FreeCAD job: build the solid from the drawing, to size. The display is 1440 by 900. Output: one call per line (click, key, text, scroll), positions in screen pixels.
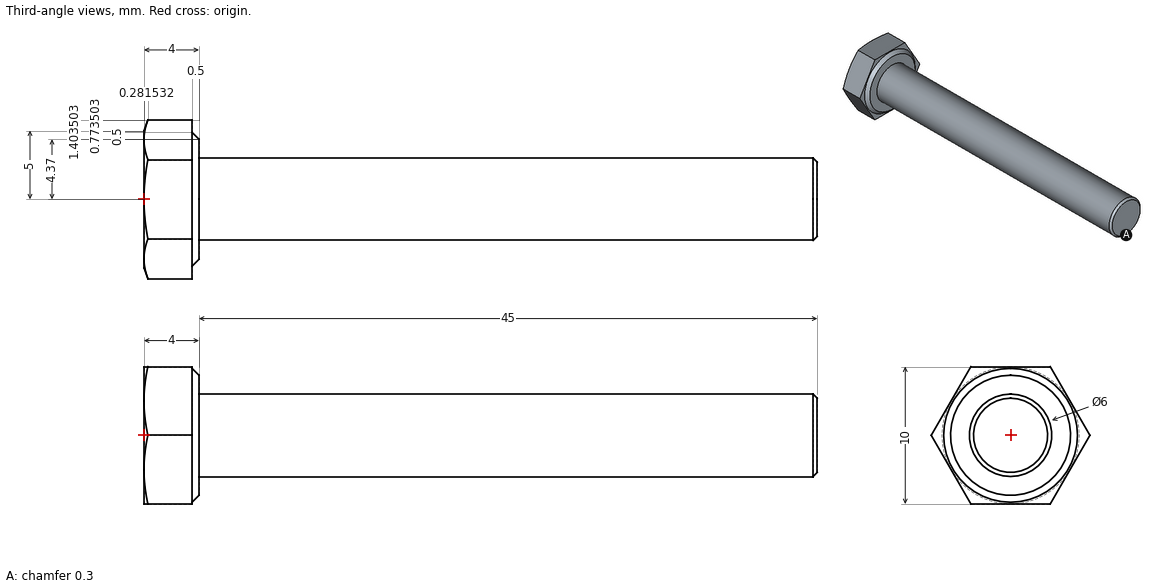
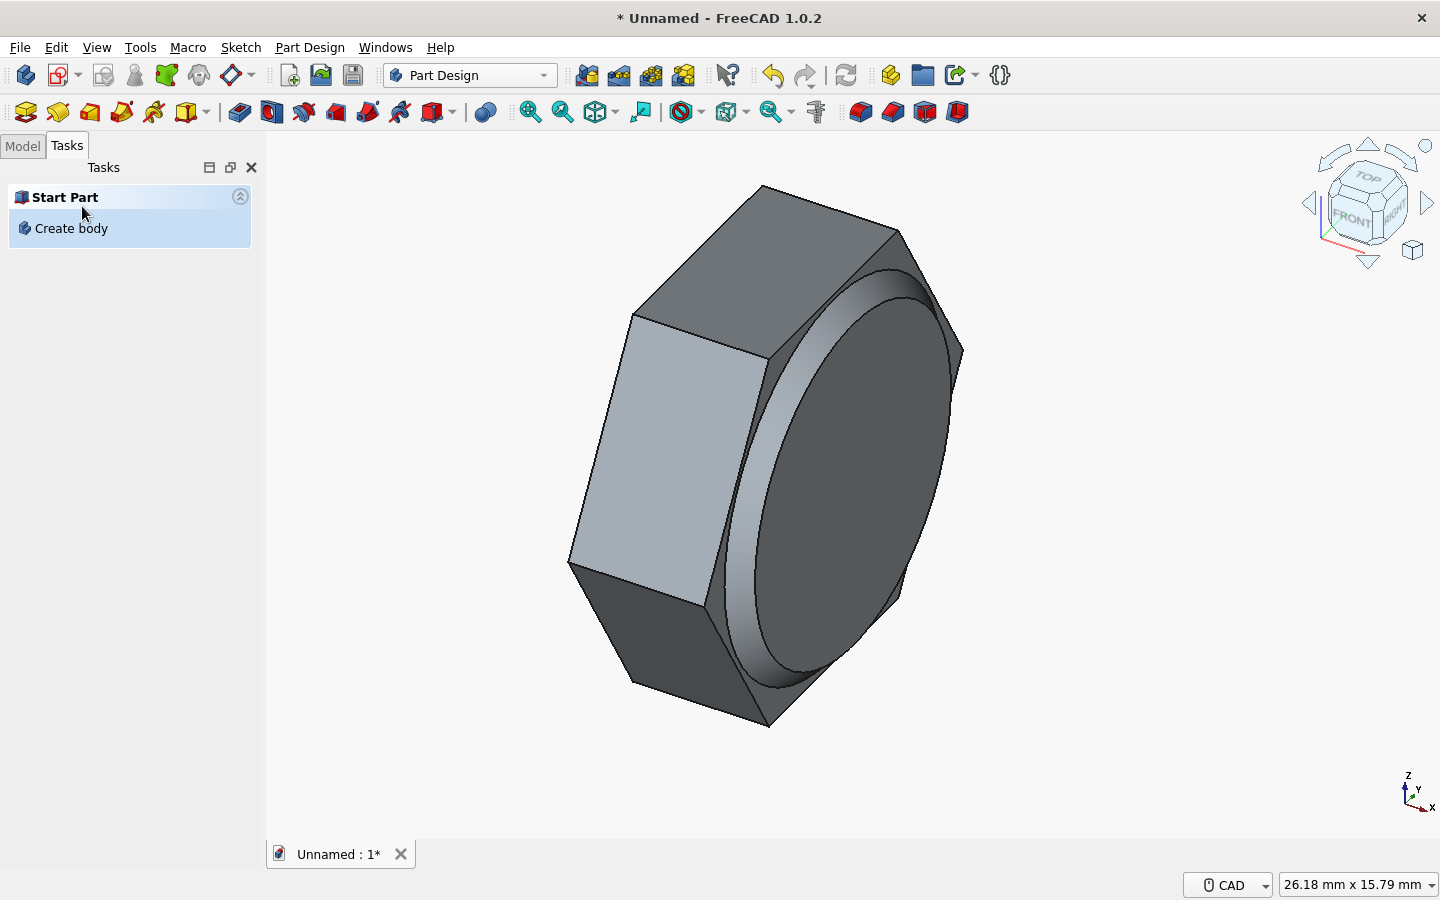
click(532, 112)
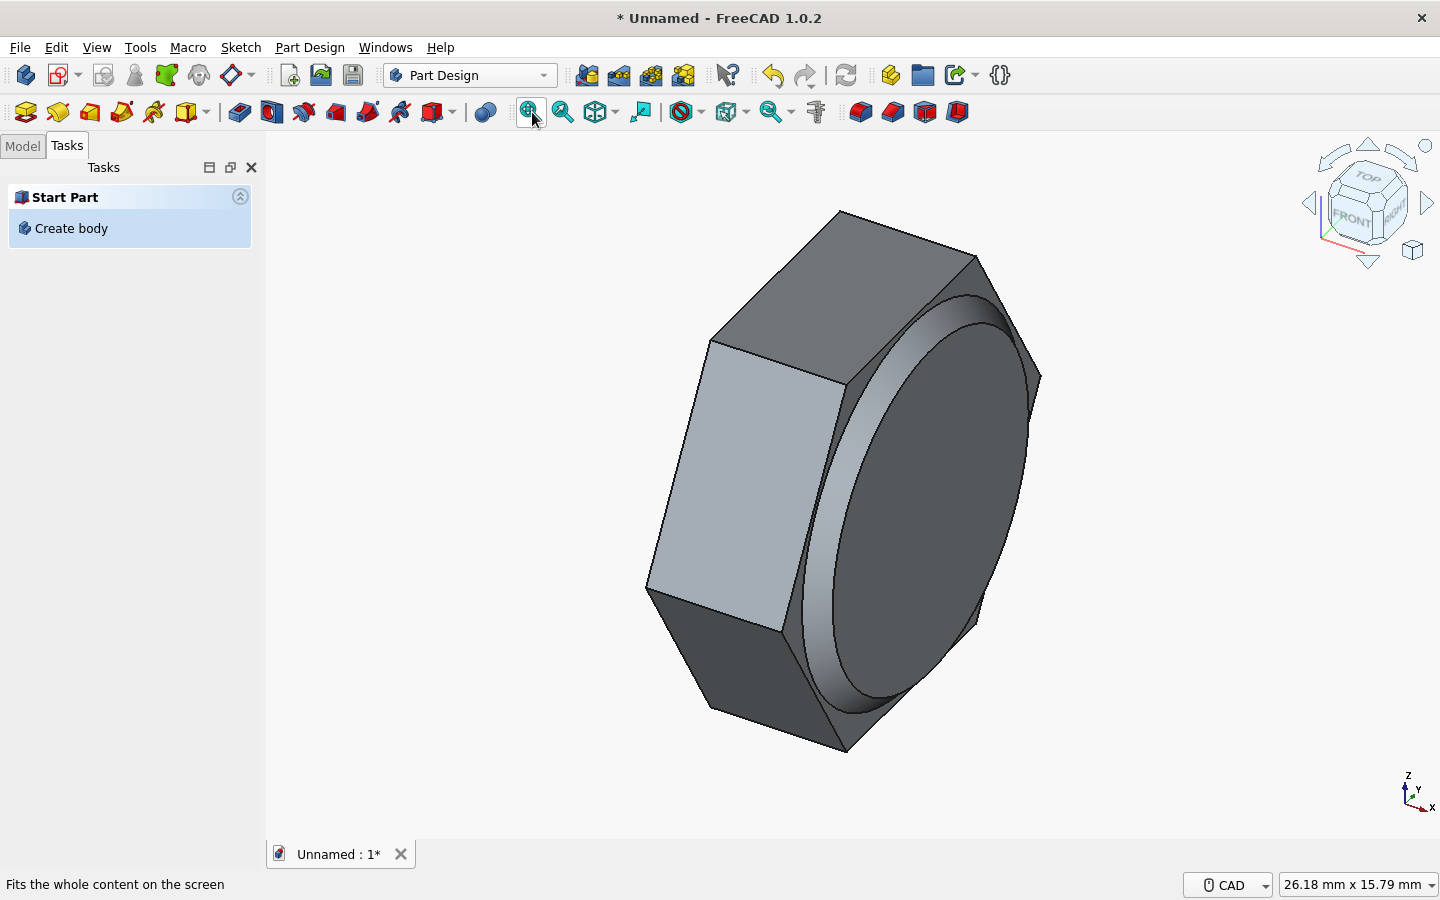
click(58, 76)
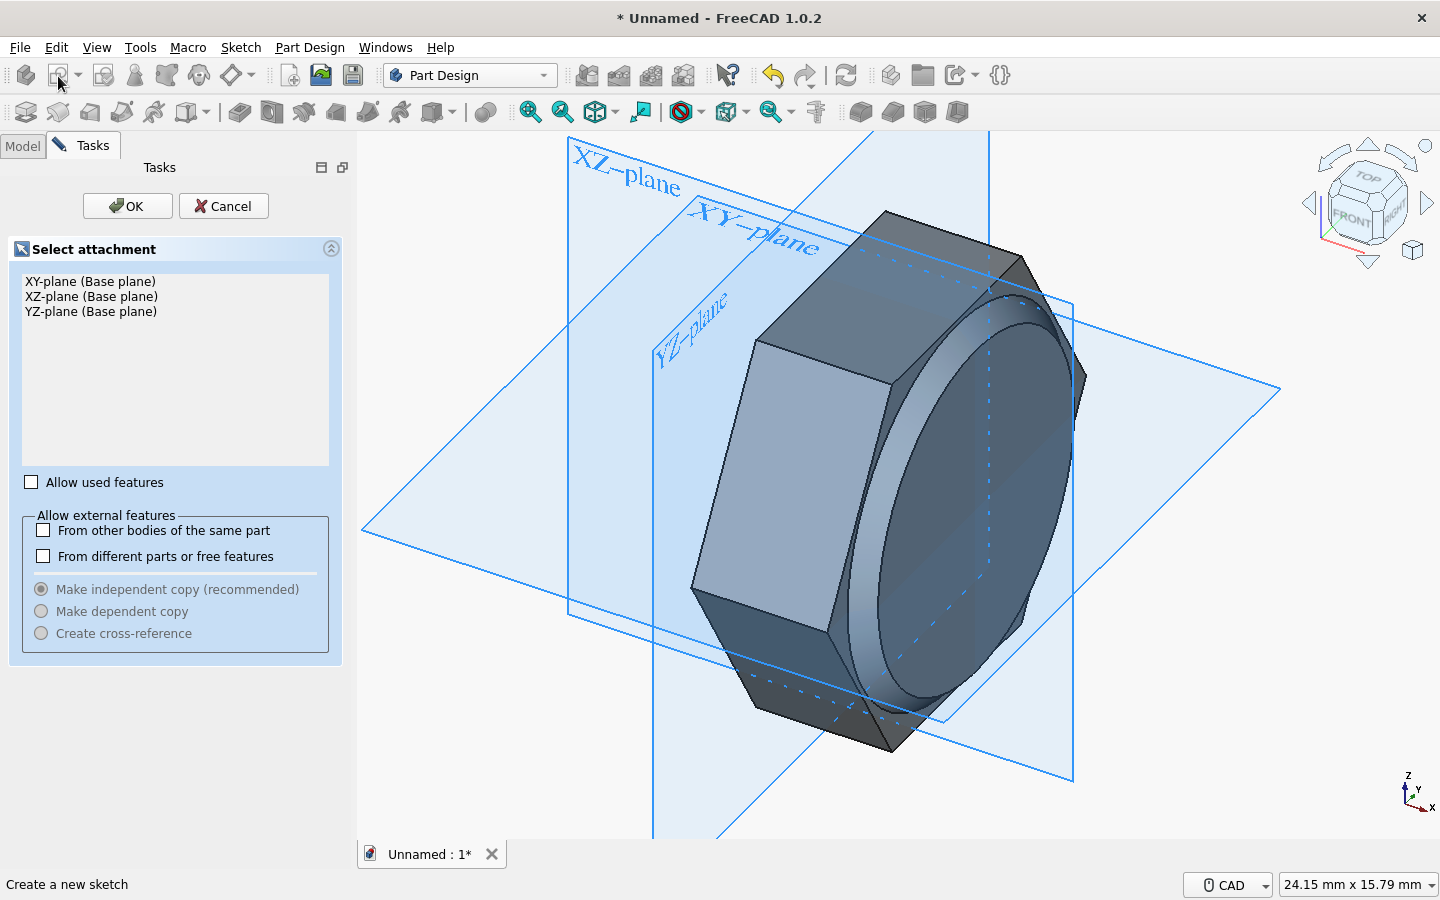
click(82, 282)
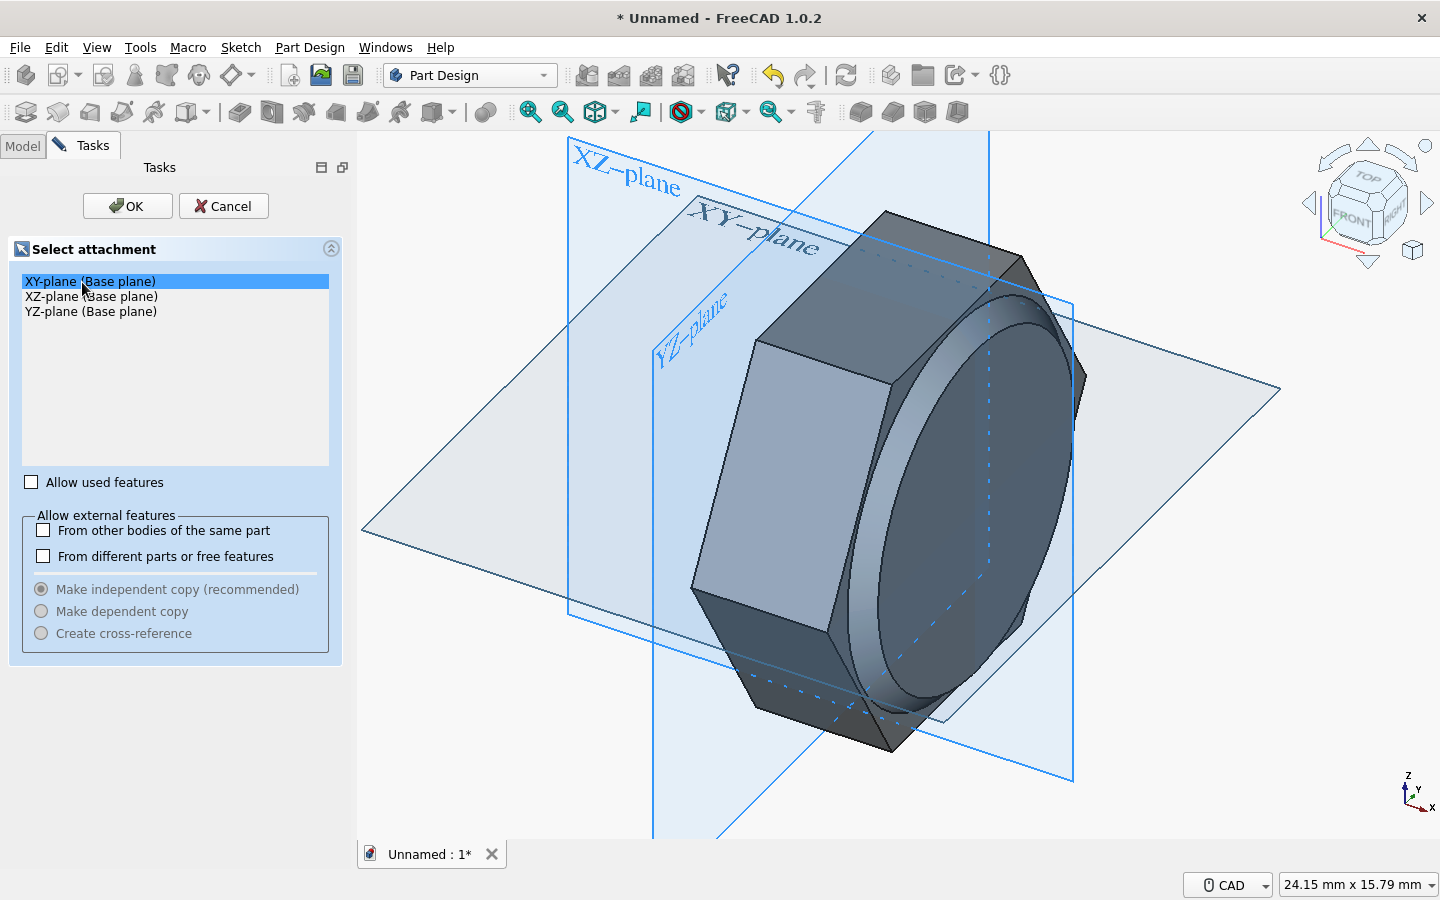
click(128, 206)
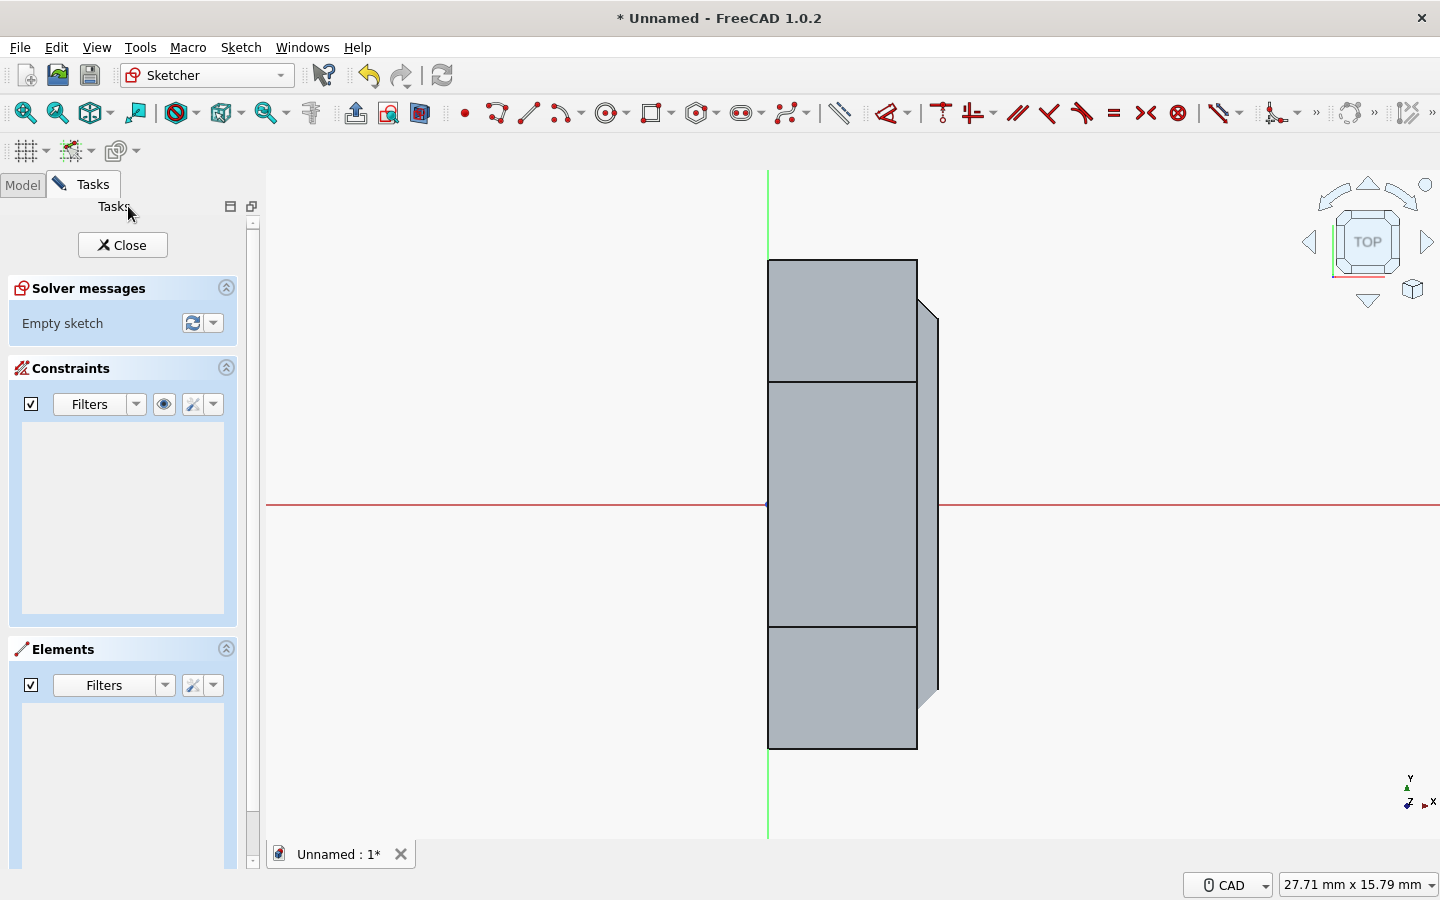
click(420, 114)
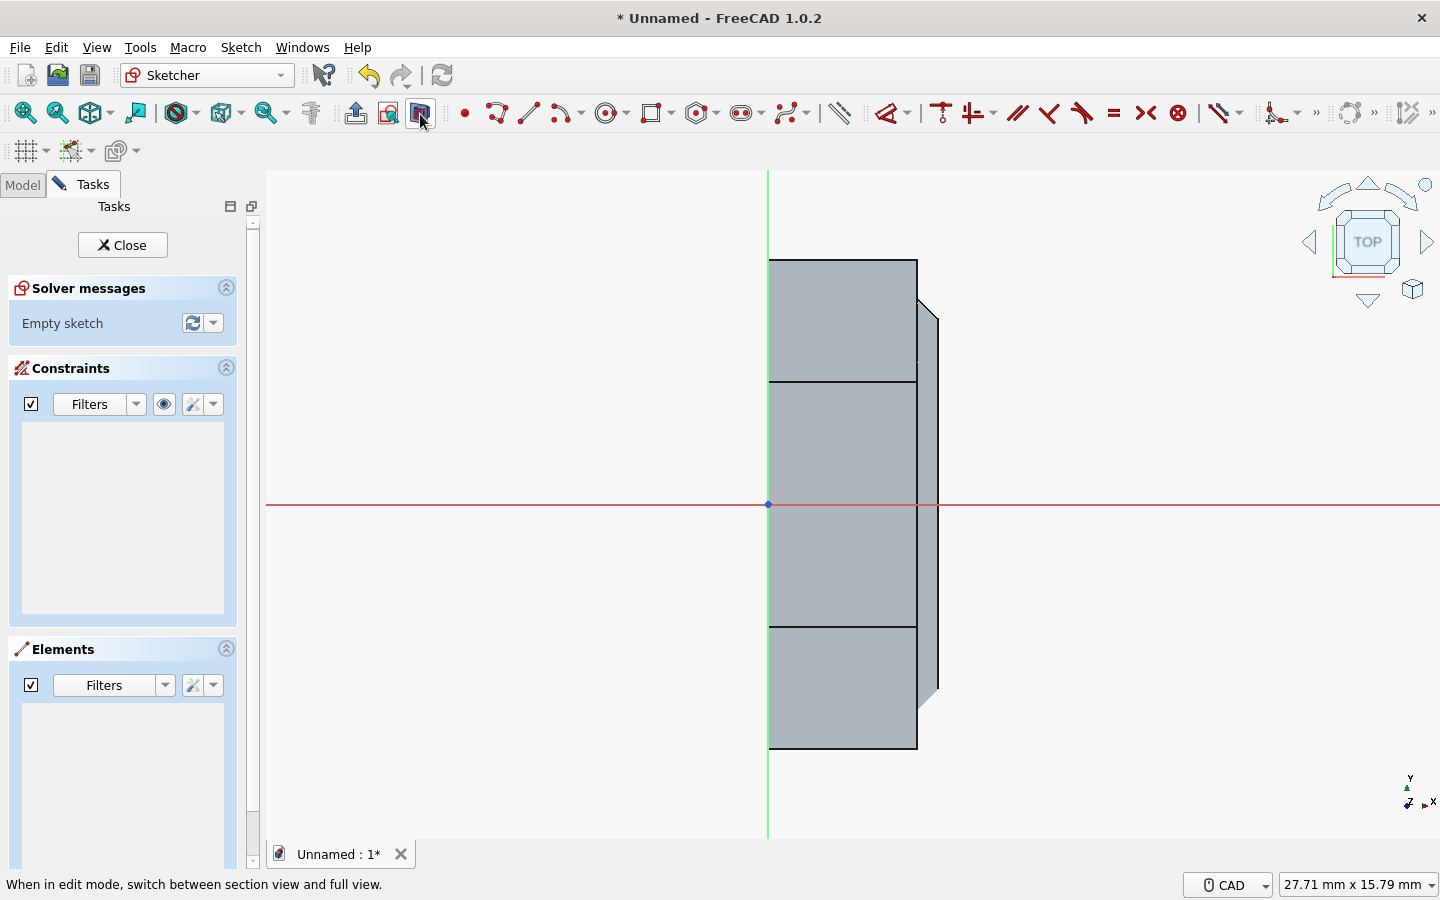
scroll(773, 258, up, 13)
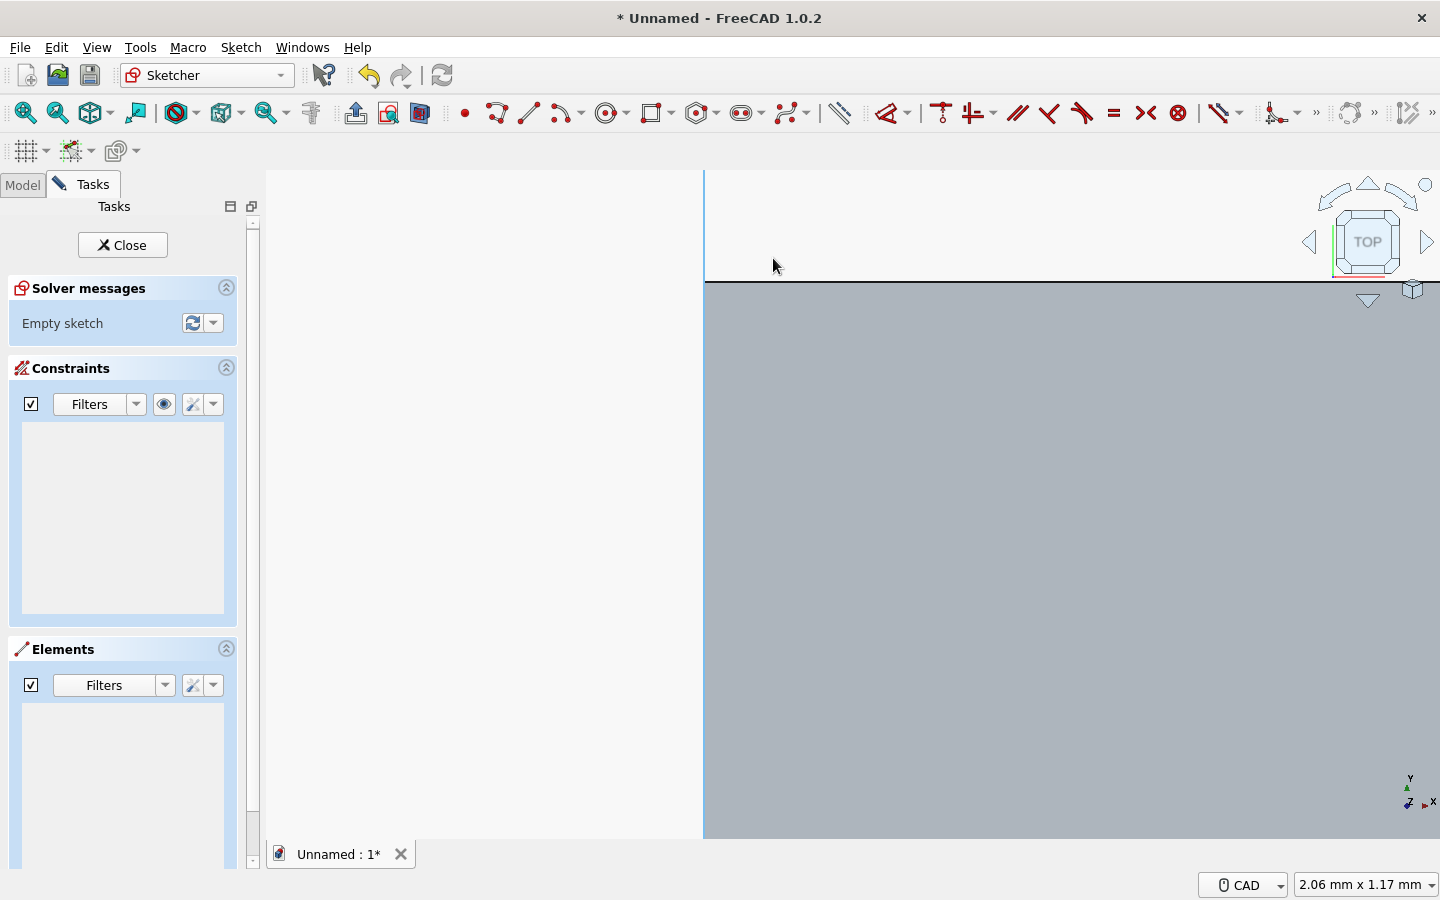
click(498, 114)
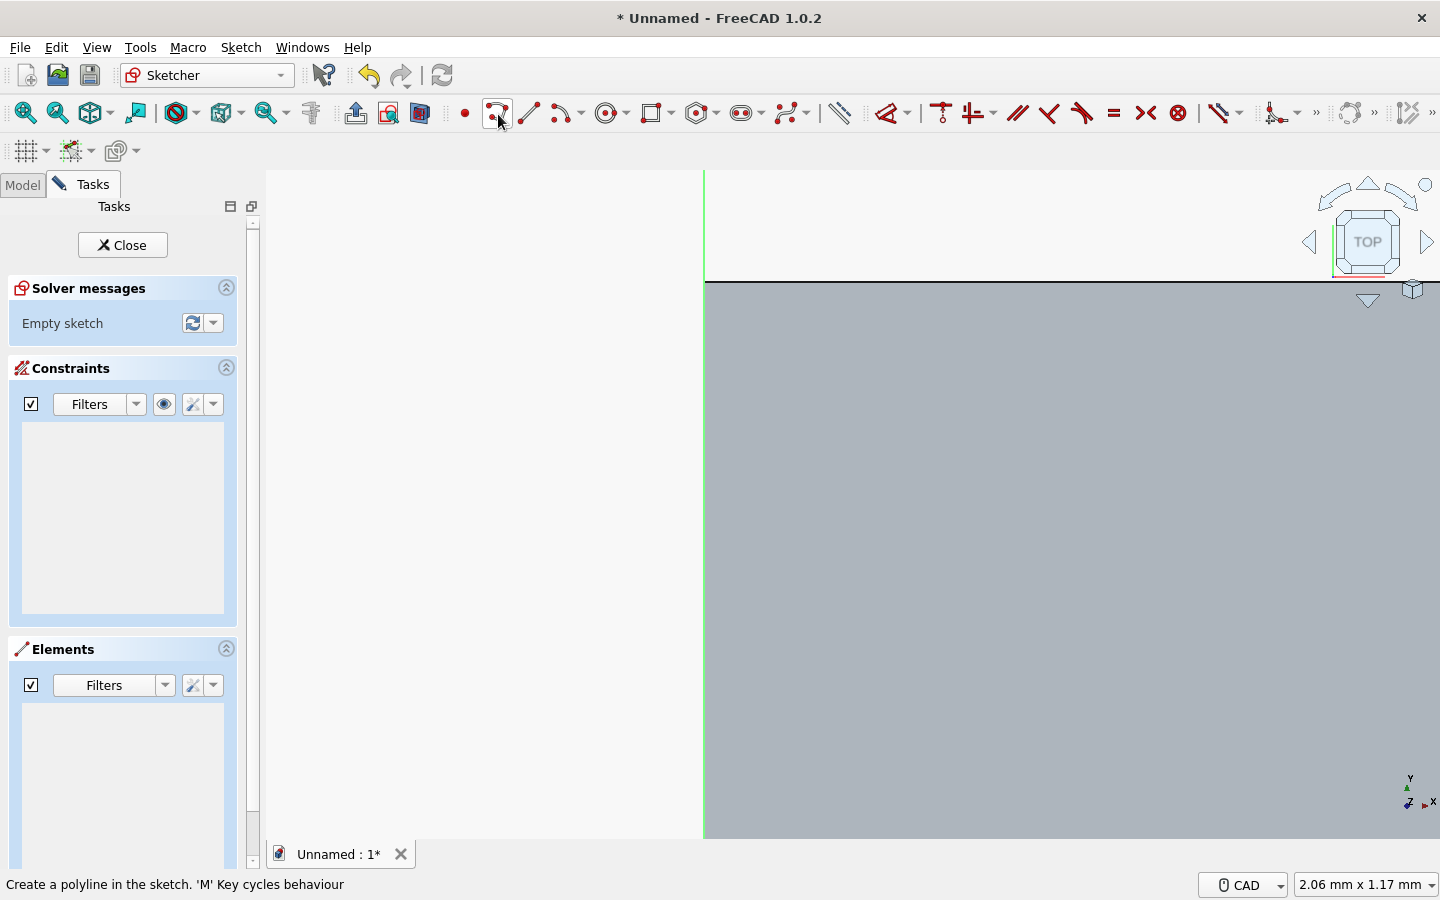
click(704, 723)
click(864, 282)
click(713, 282)
click(704, 724)
key(Escape)
key(Escape)